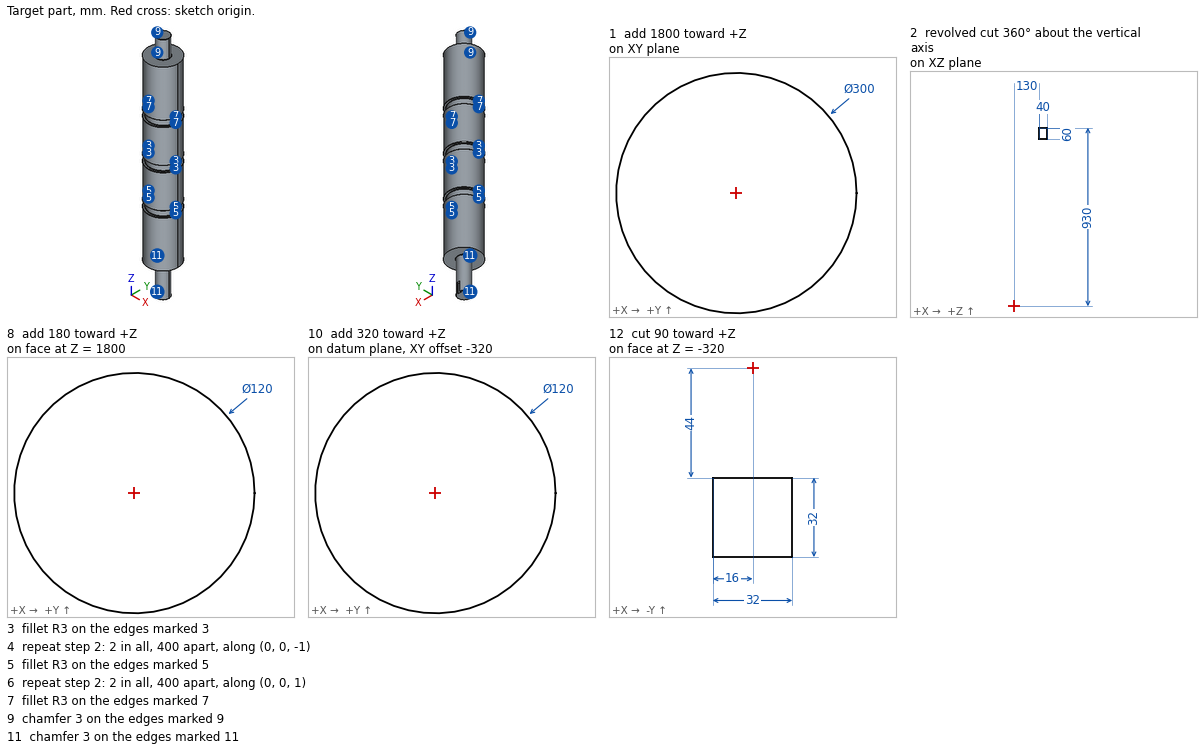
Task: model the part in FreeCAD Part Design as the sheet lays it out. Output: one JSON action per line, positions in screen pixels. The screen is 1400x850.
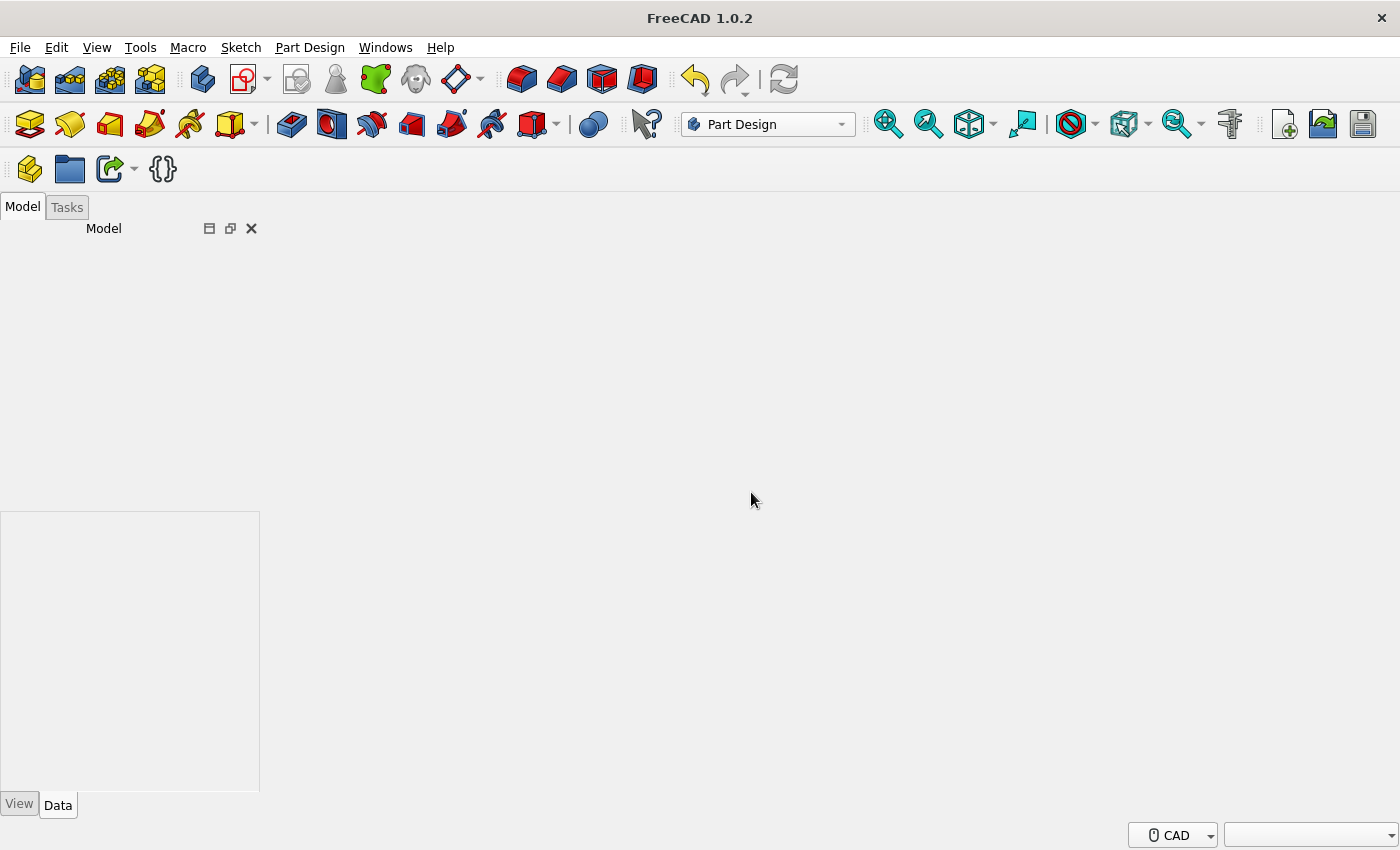
{"action": "left_click", "coordinate": [1284, 124]}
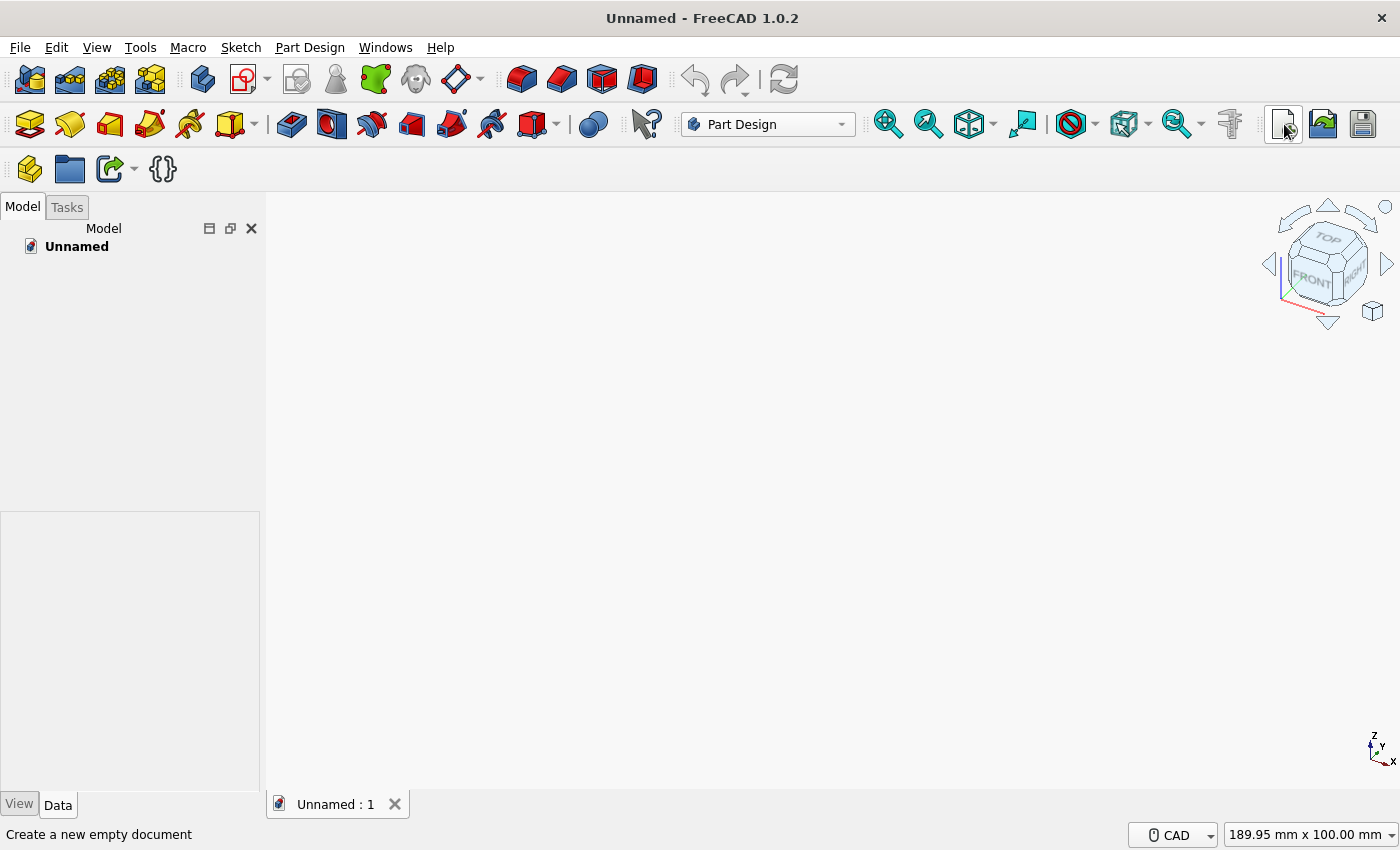
{"action": "left_click", "coordinate": [244, 80]}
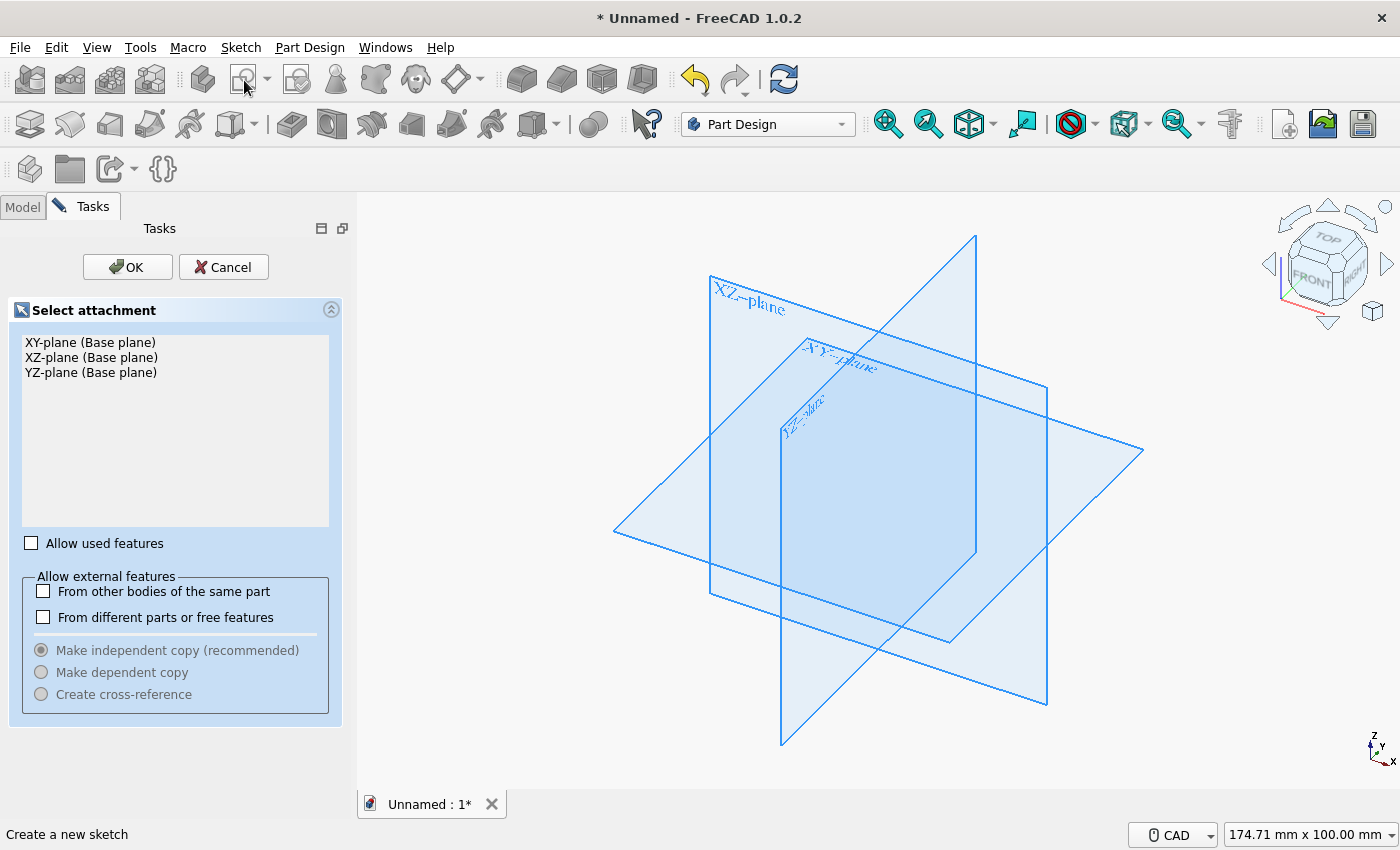
{"action": "left_click", "coordinate": [82, 342]}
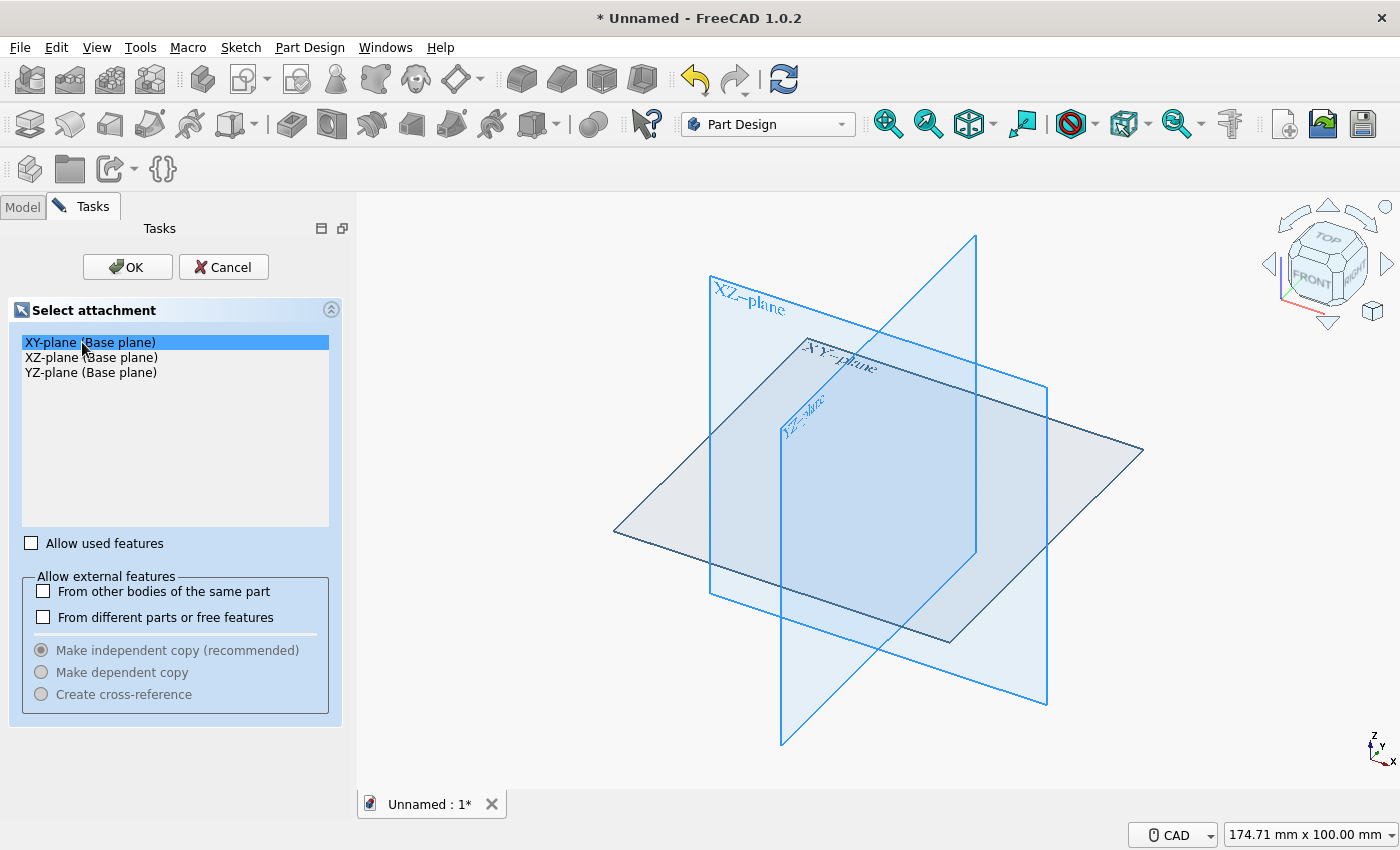
{"action": "left_click", "coordinate": [128, 267]}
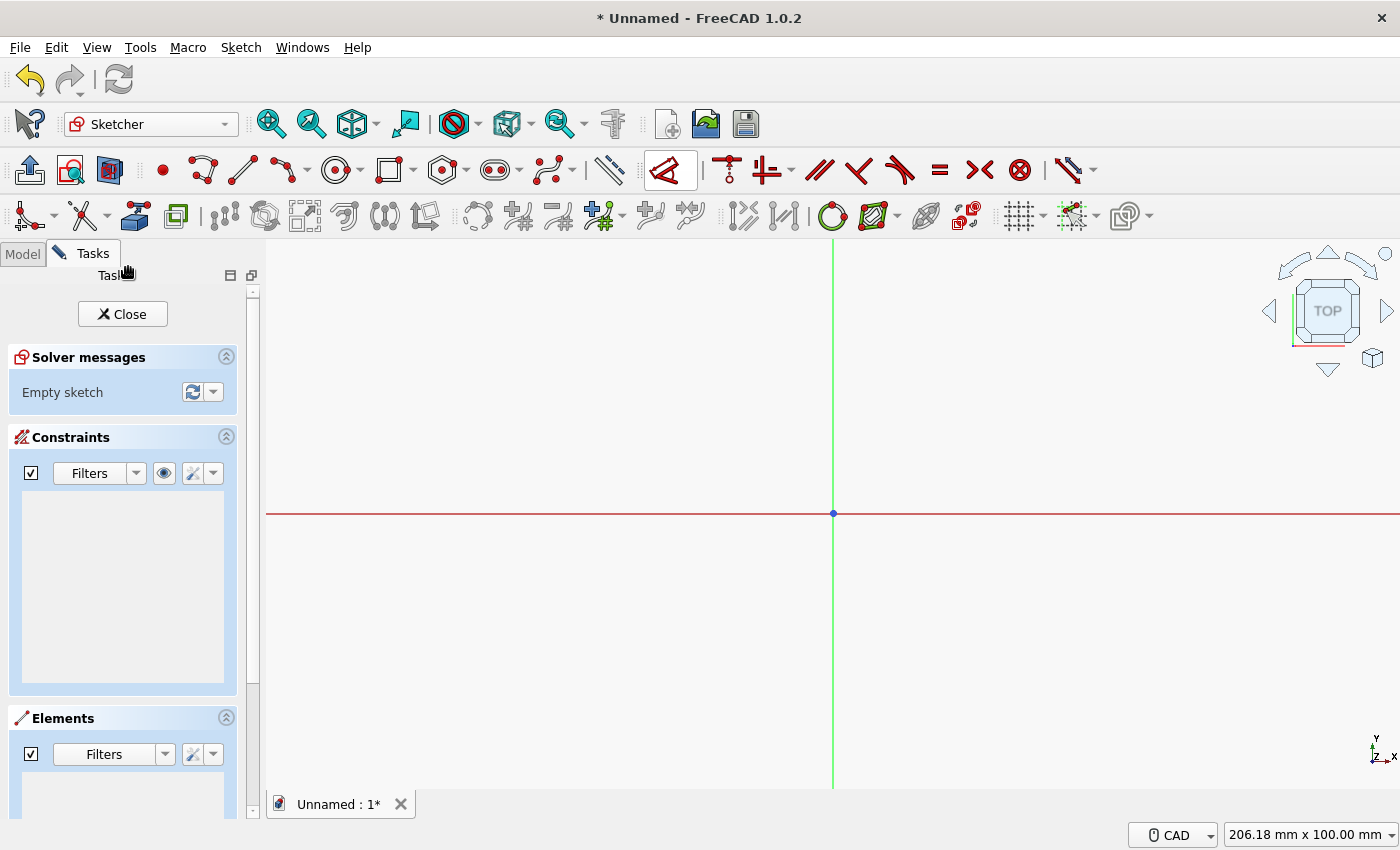
{"action": "scroll", "coordinate": [747, 514], "scroll_direction": "down", "scroll_amount": 8}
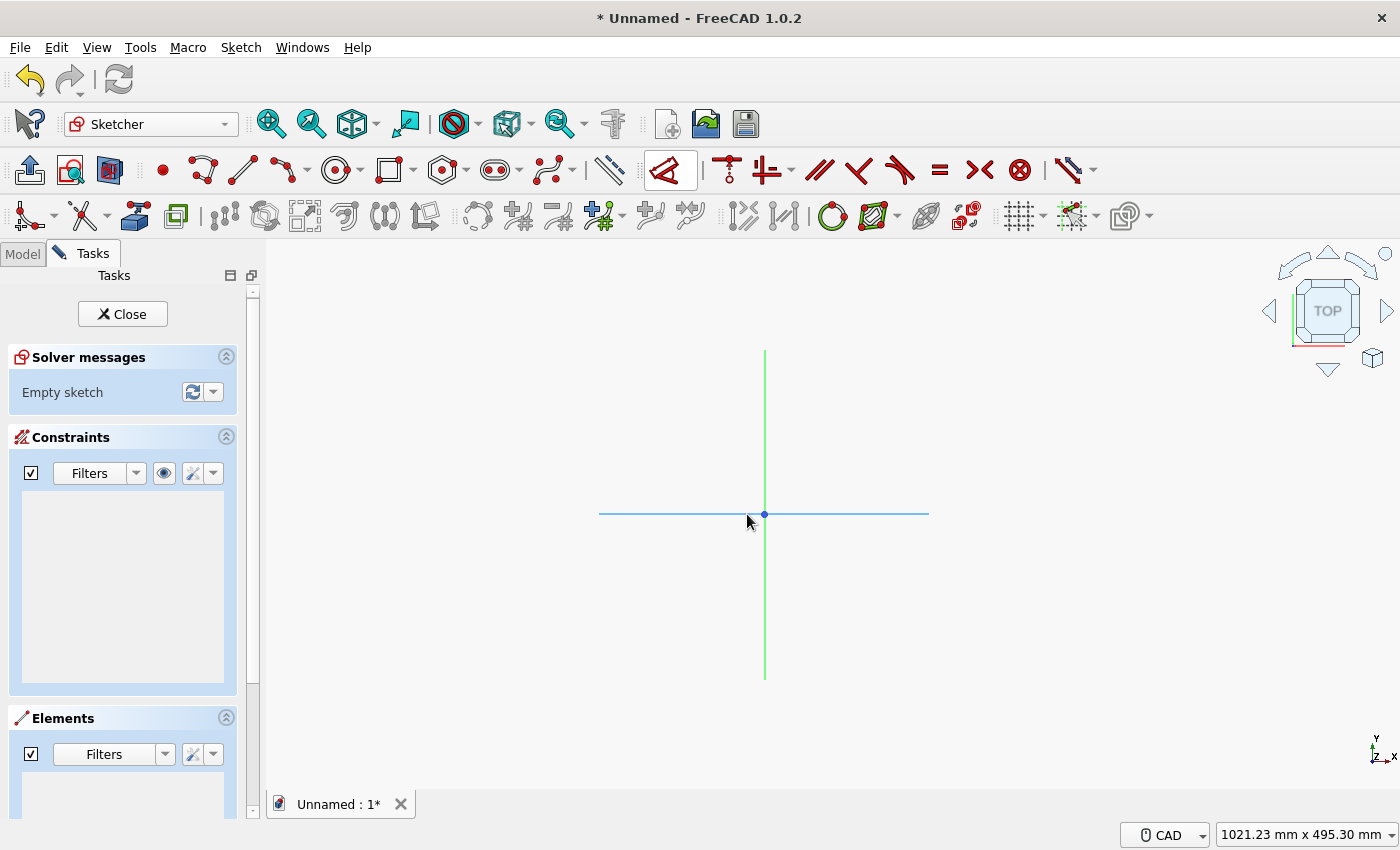
{"action": "left_click", "coordinate": [336, 170]}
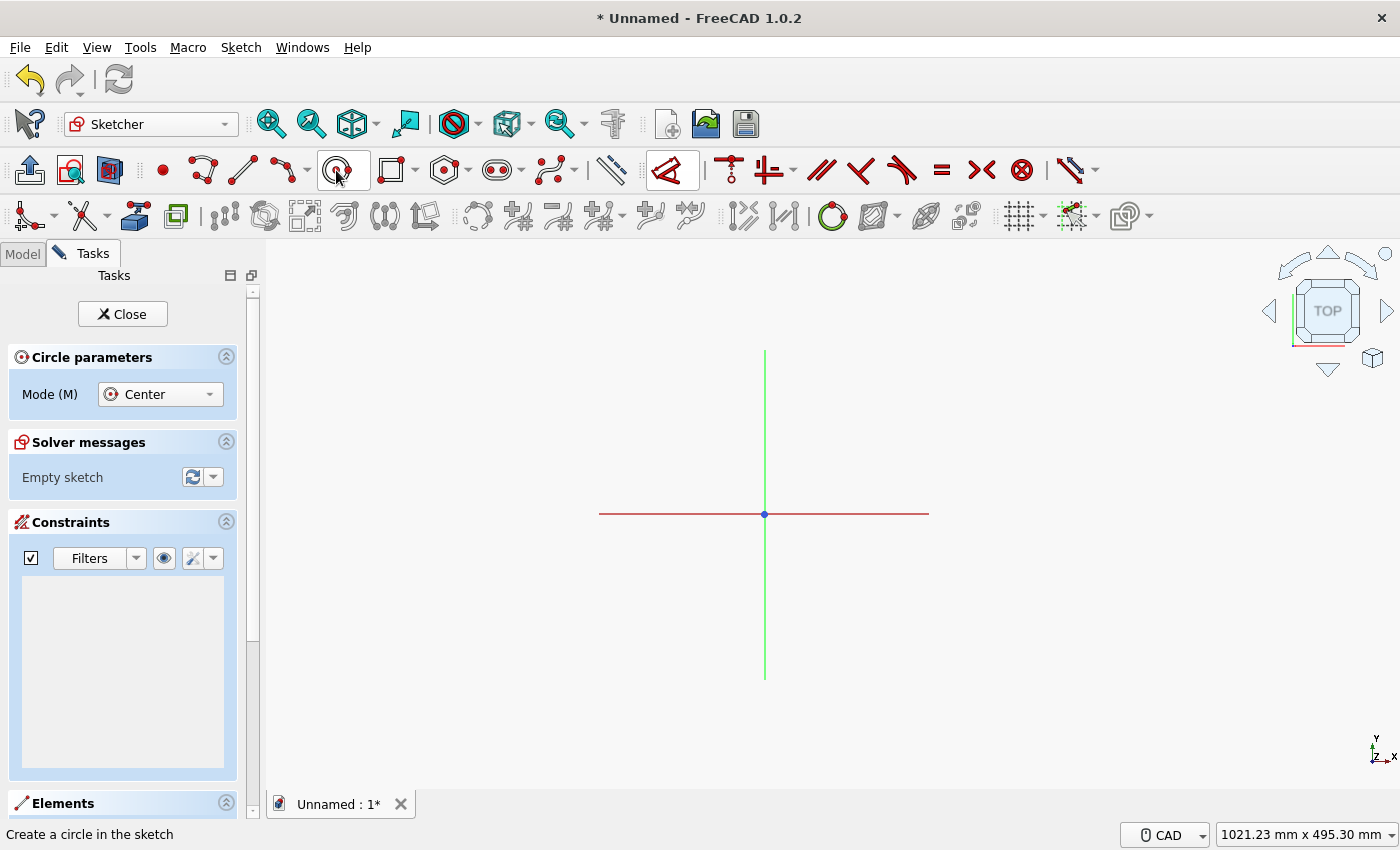
{"action": "left_click", "coordinate": [765, 514]}
{"action": "mouse_move", "coordinate": [882, 397]}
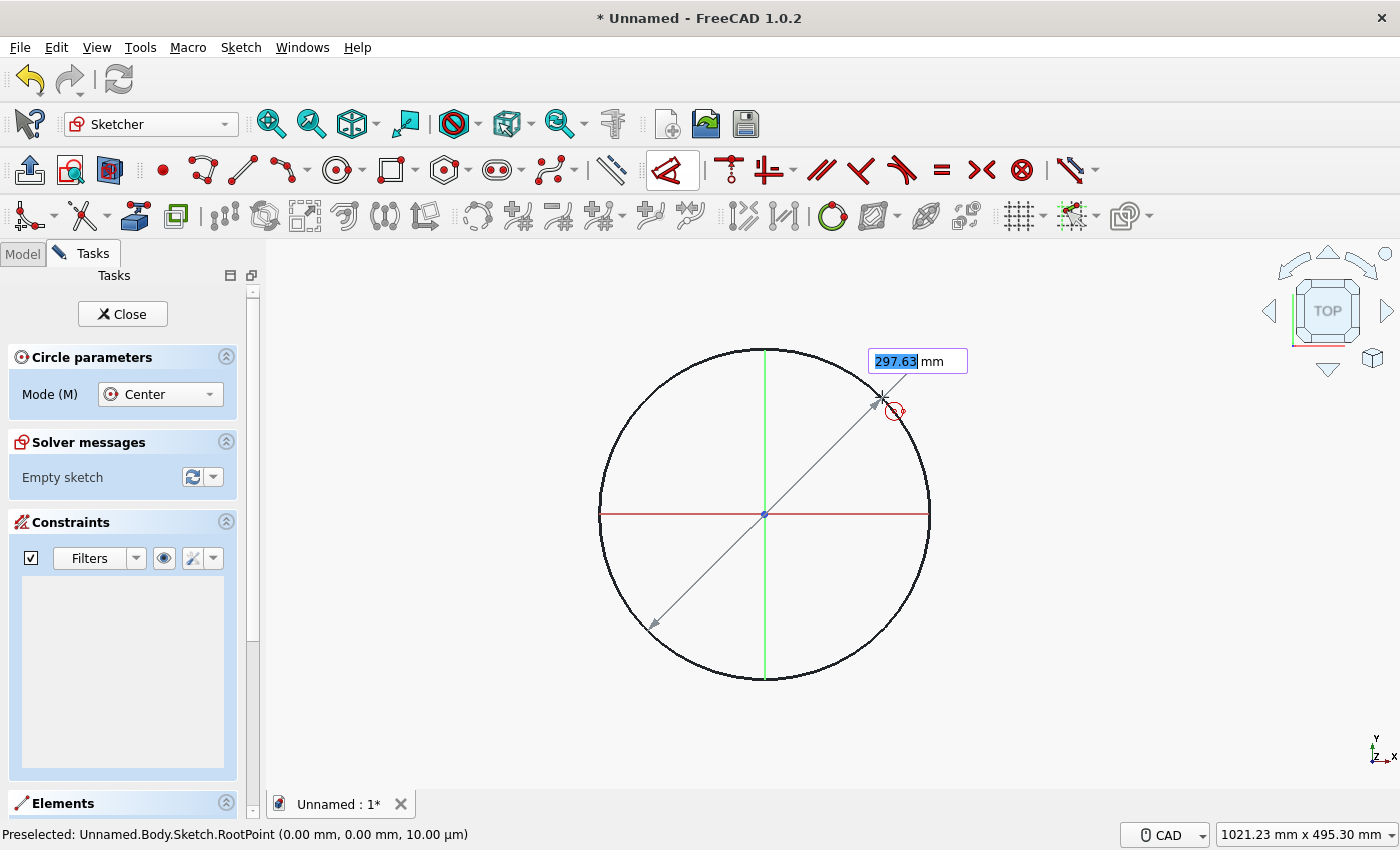
{"action": "type", "text": "300"}
{"action": "key", "text": "Return"}
{"action": "key", "text": "Escape"}